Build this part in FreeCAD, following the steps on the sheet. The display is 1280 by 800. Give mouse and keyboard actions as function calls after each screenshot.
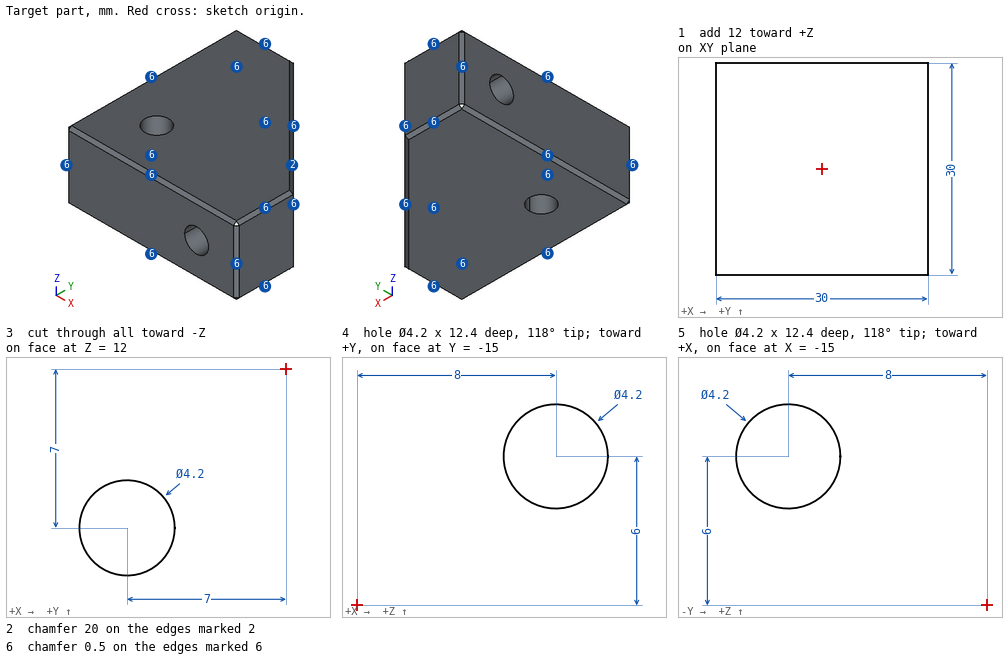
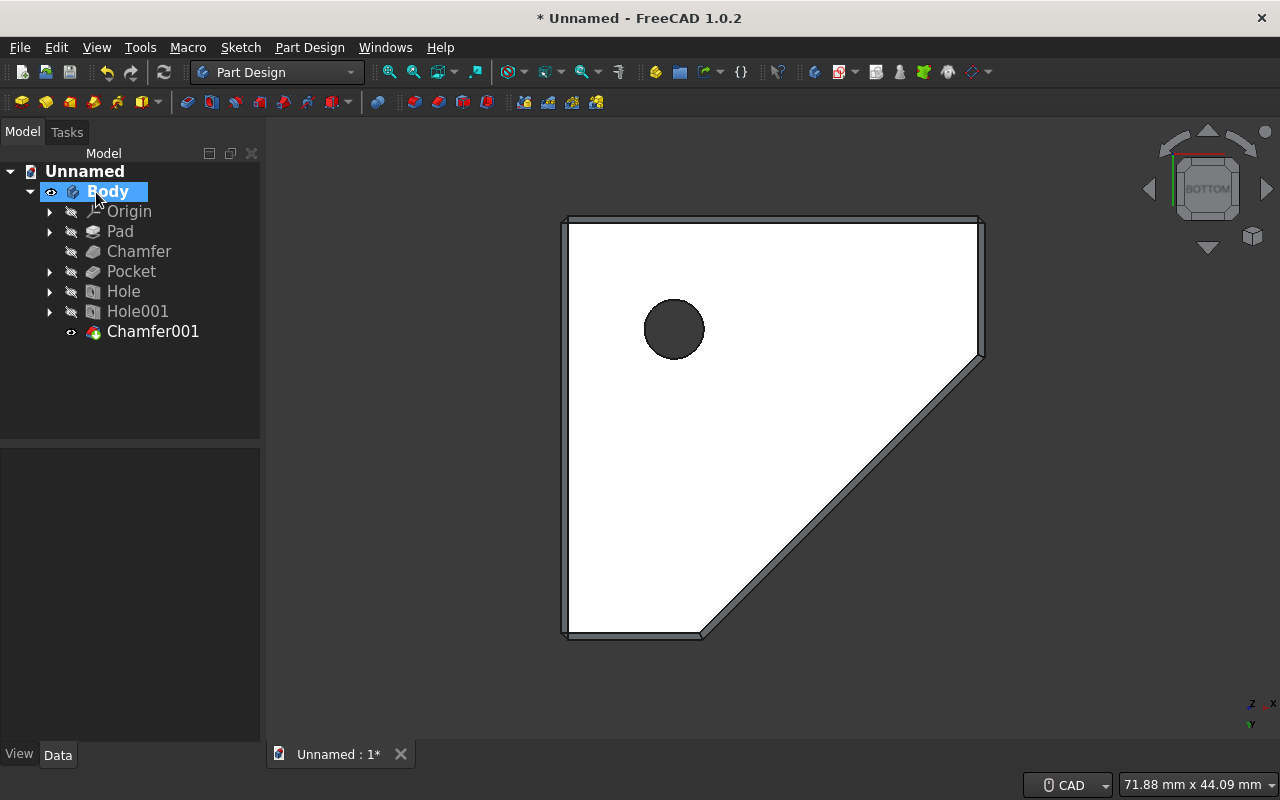
key(0)